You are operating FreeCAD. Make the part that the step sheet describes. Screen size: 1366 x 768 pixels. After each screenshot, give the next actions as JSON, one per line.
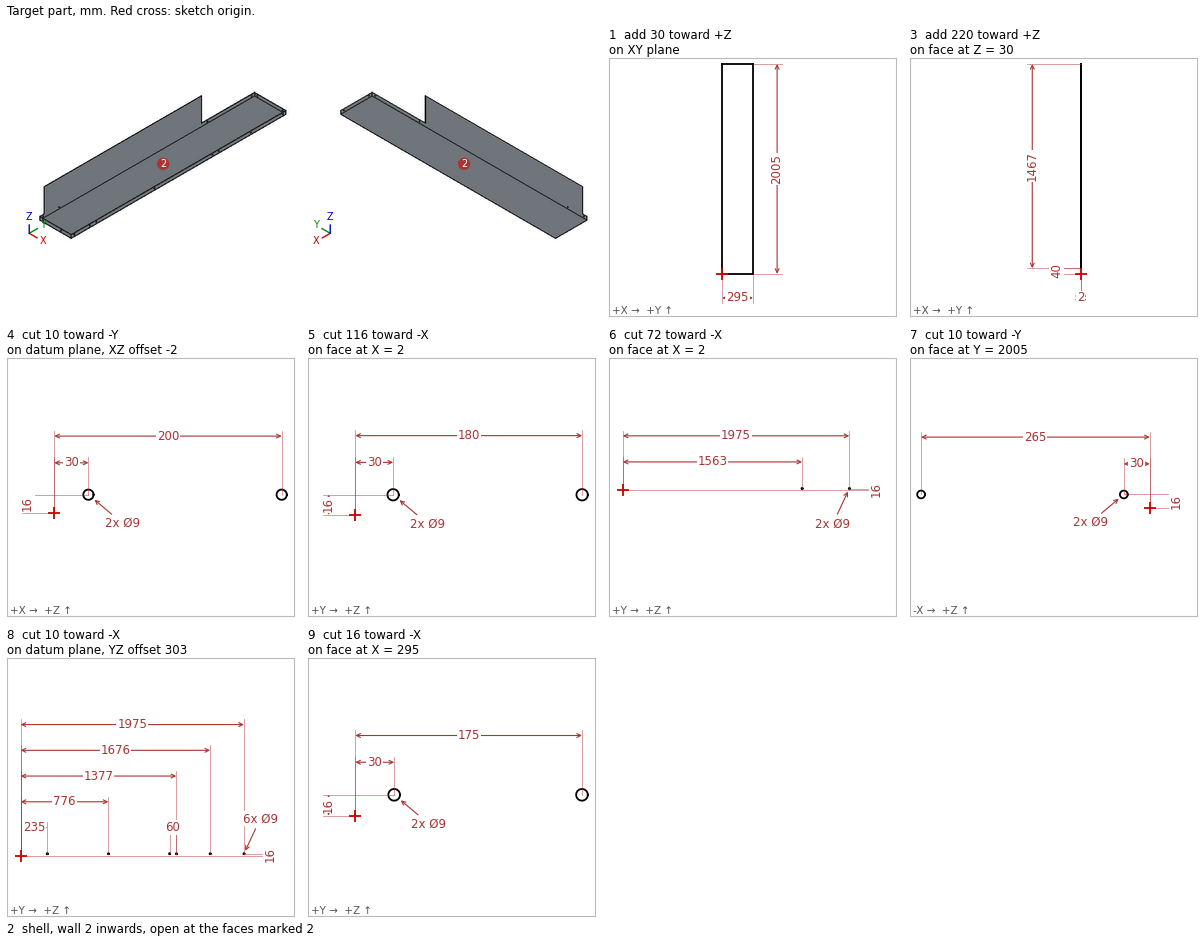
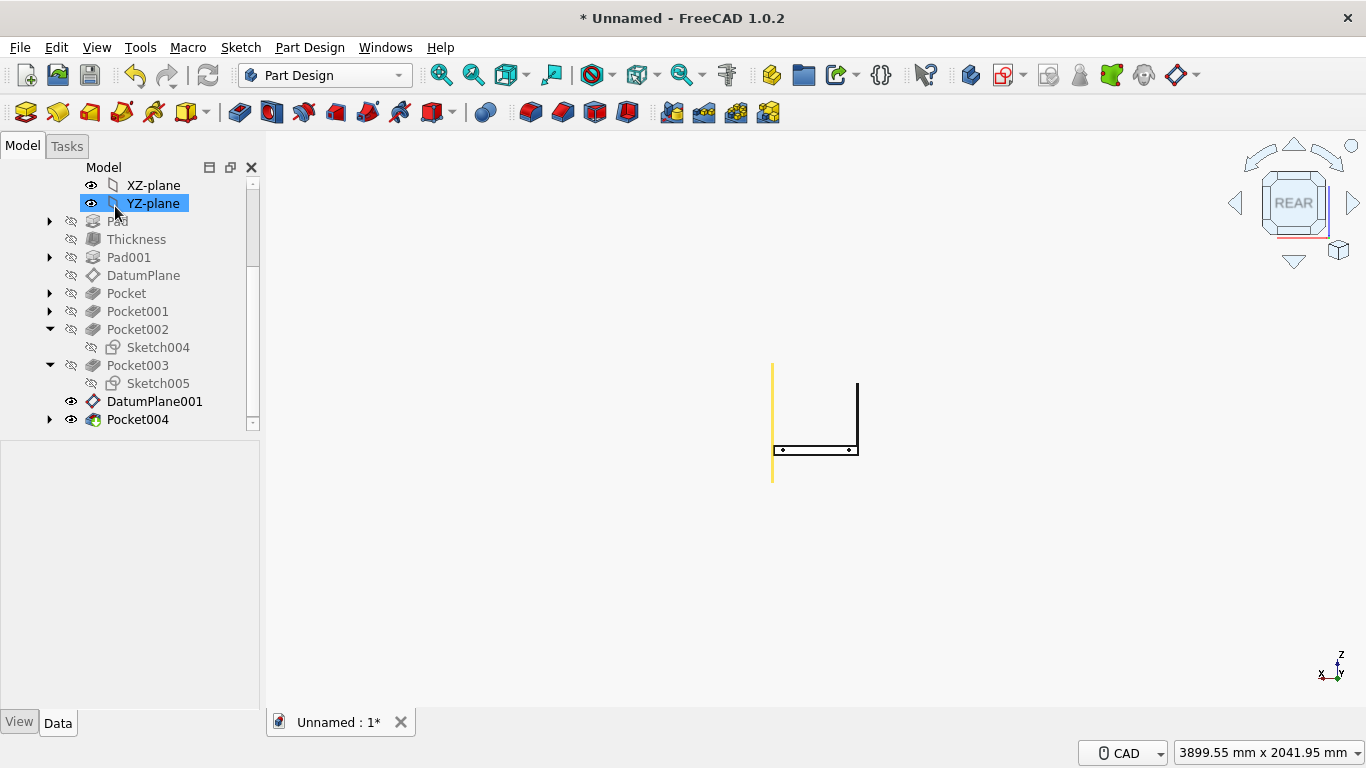
{"action": "left_click", "coordinate": [116, 401]}
{"action": "key", "text": "space"}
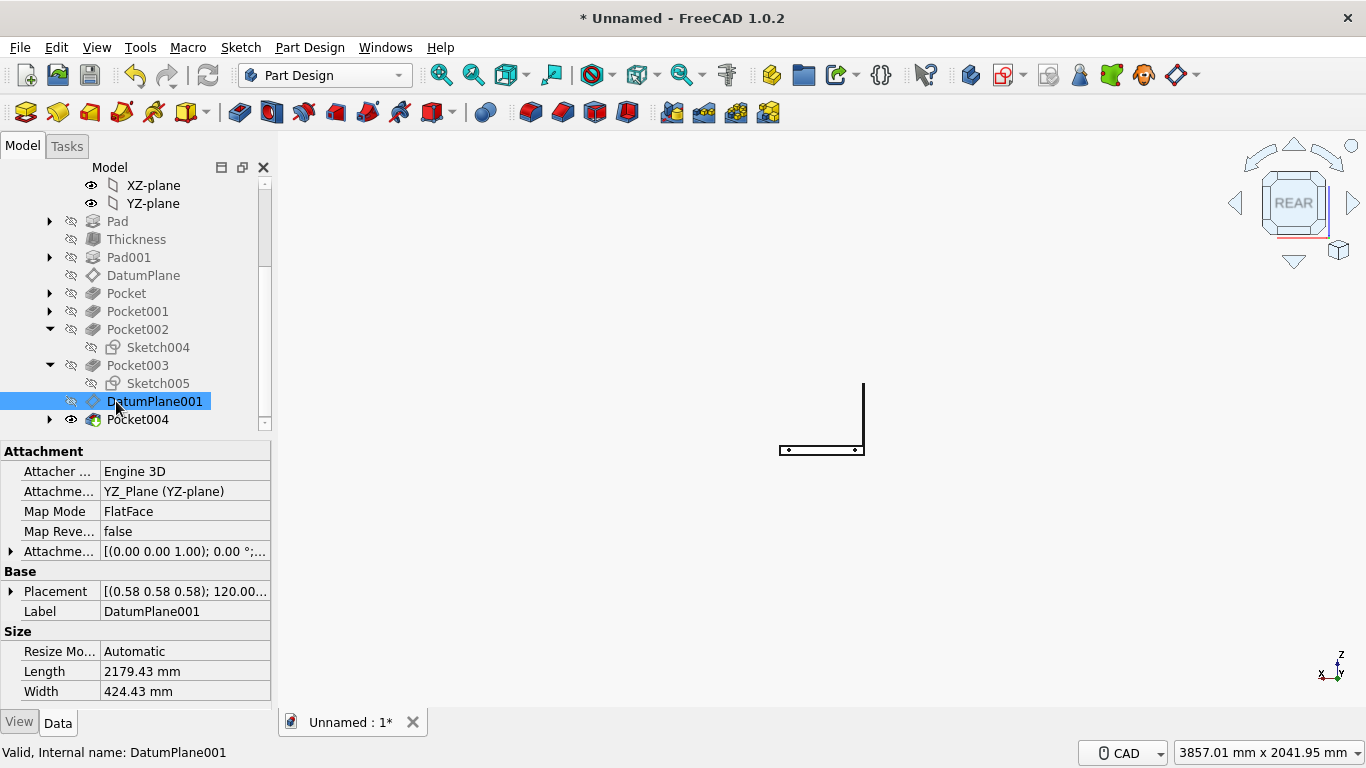
{"action": "key", "text": "v f"}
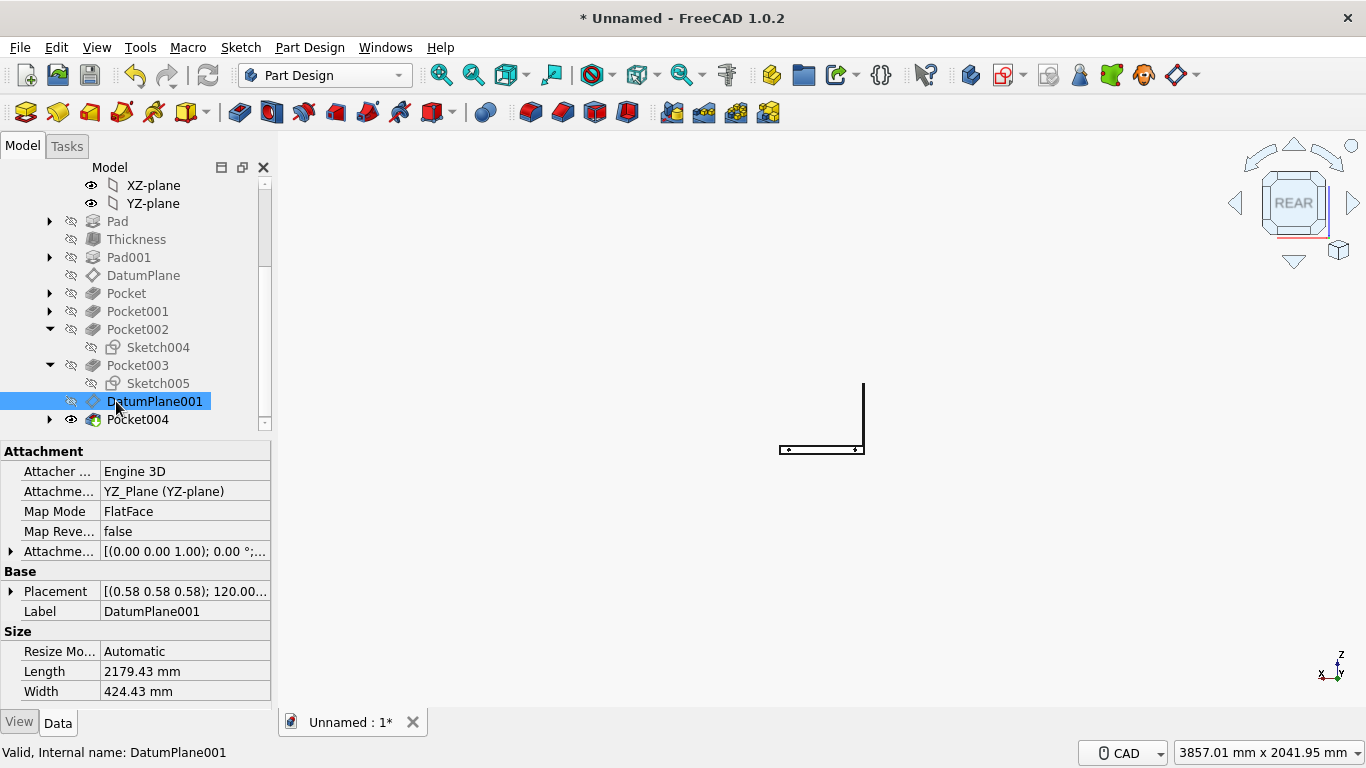
{"action": "key", "text": "0"}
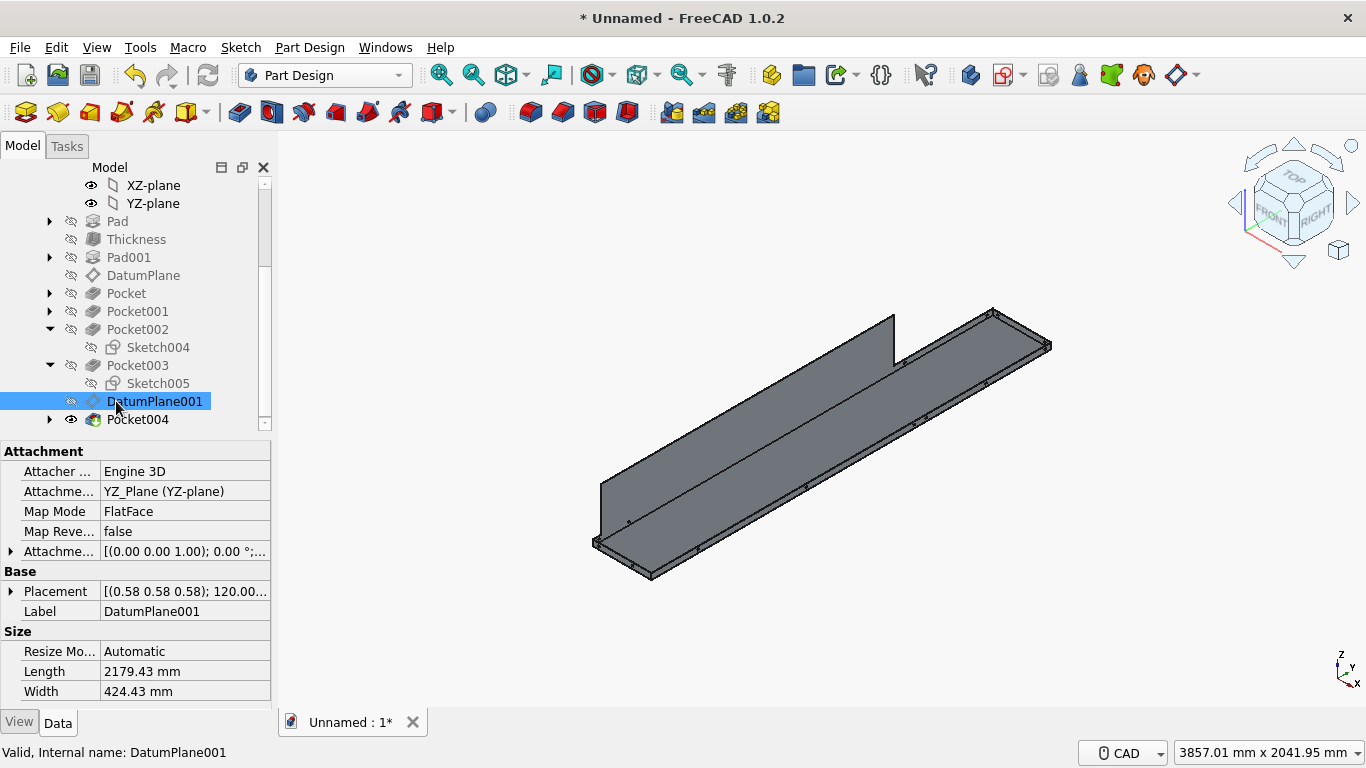
{"action": "scroll", "coordinate": [1023, 361], "scroll_direction": "up", "scroll_amount": 6}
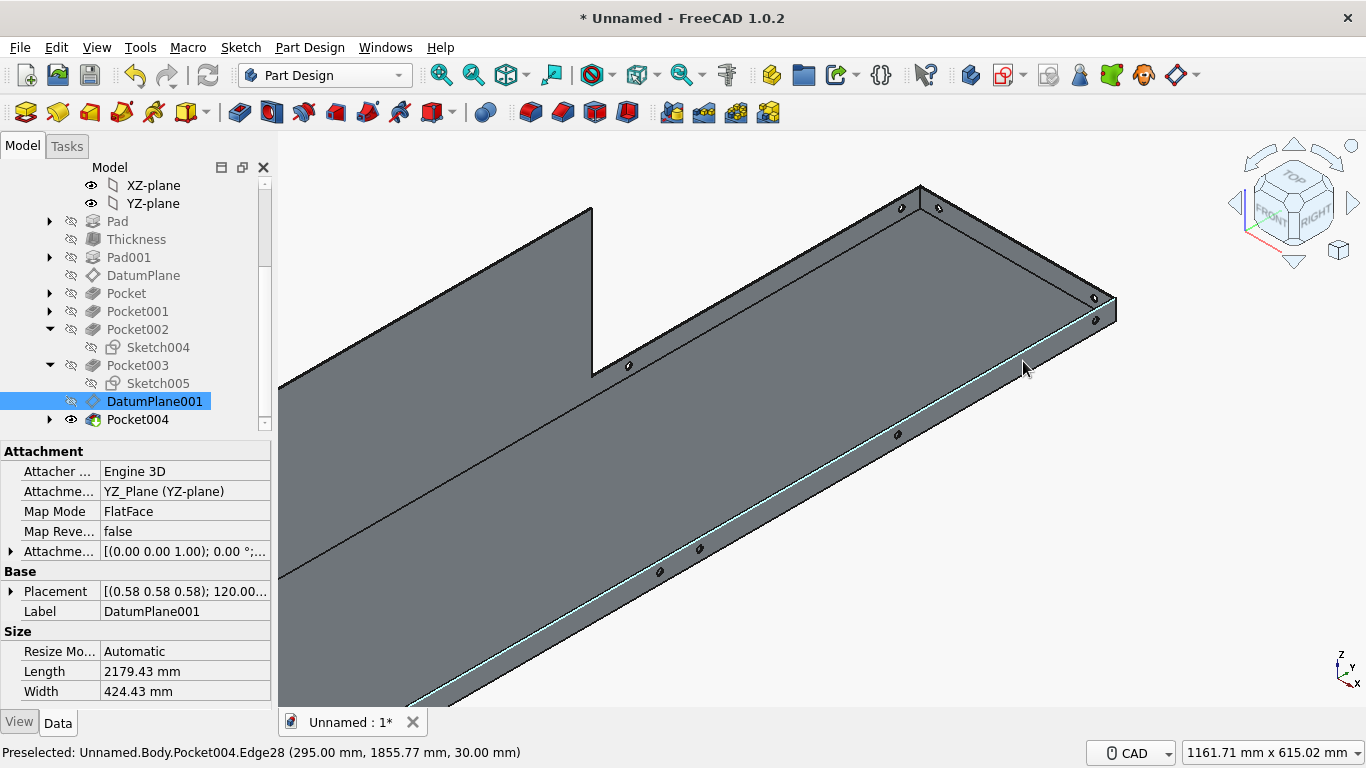
{"action": "left_click", "coordinate": [1021, 364]}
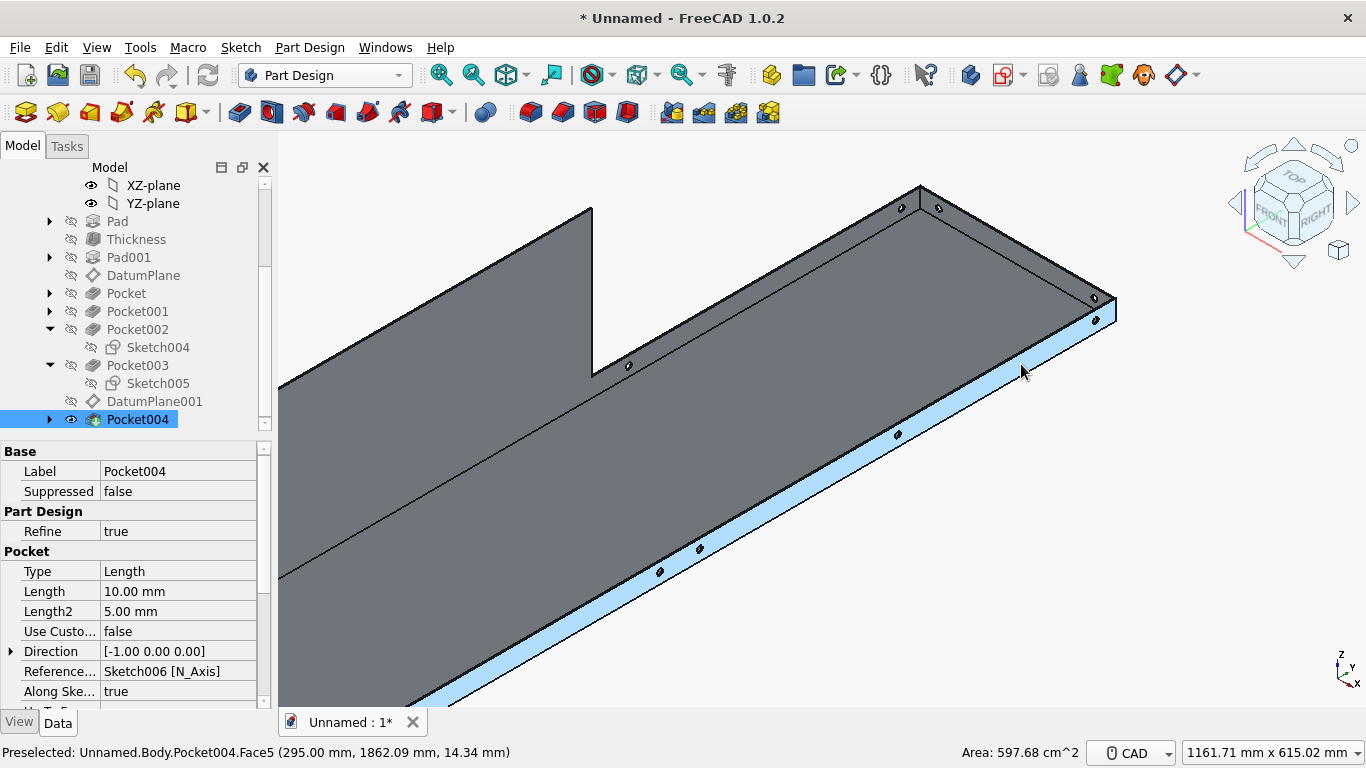
{"action": "left_click", "coordinate": [1004, 76]}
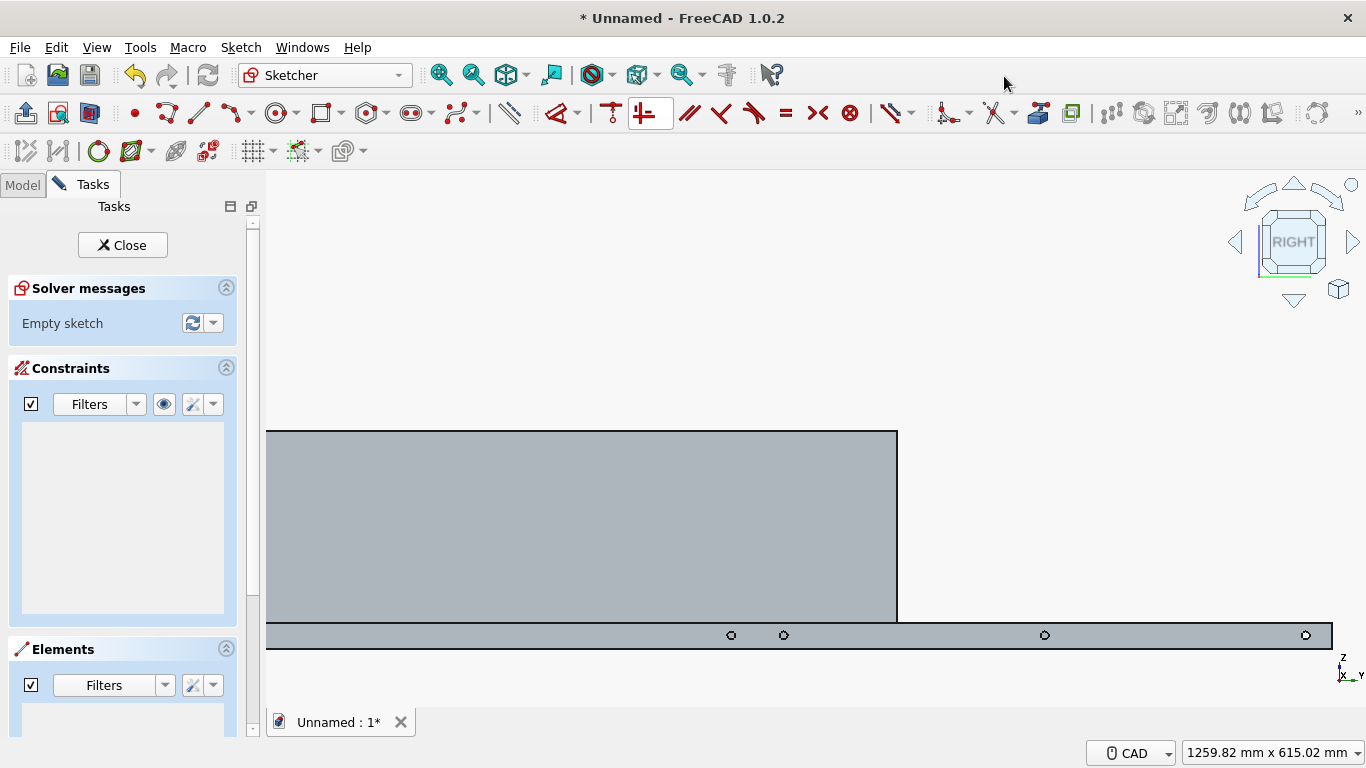
{"action": "scroll", "coordinate": [748, 438], "scroll_direction": "down", "scroll_amount": 5}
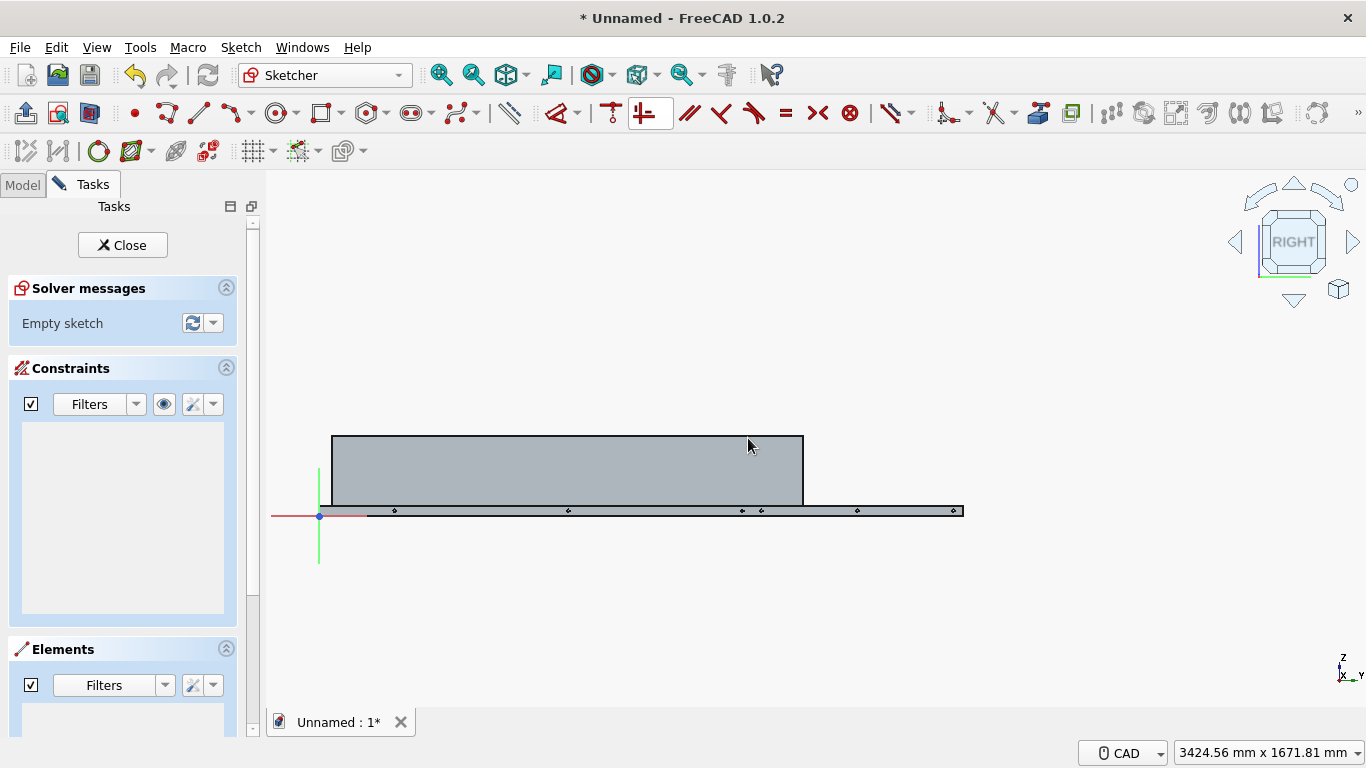
{"action": "scroll", "coordinate": [308, 520], "scroll_direction": "up", "scroll_amount": 12}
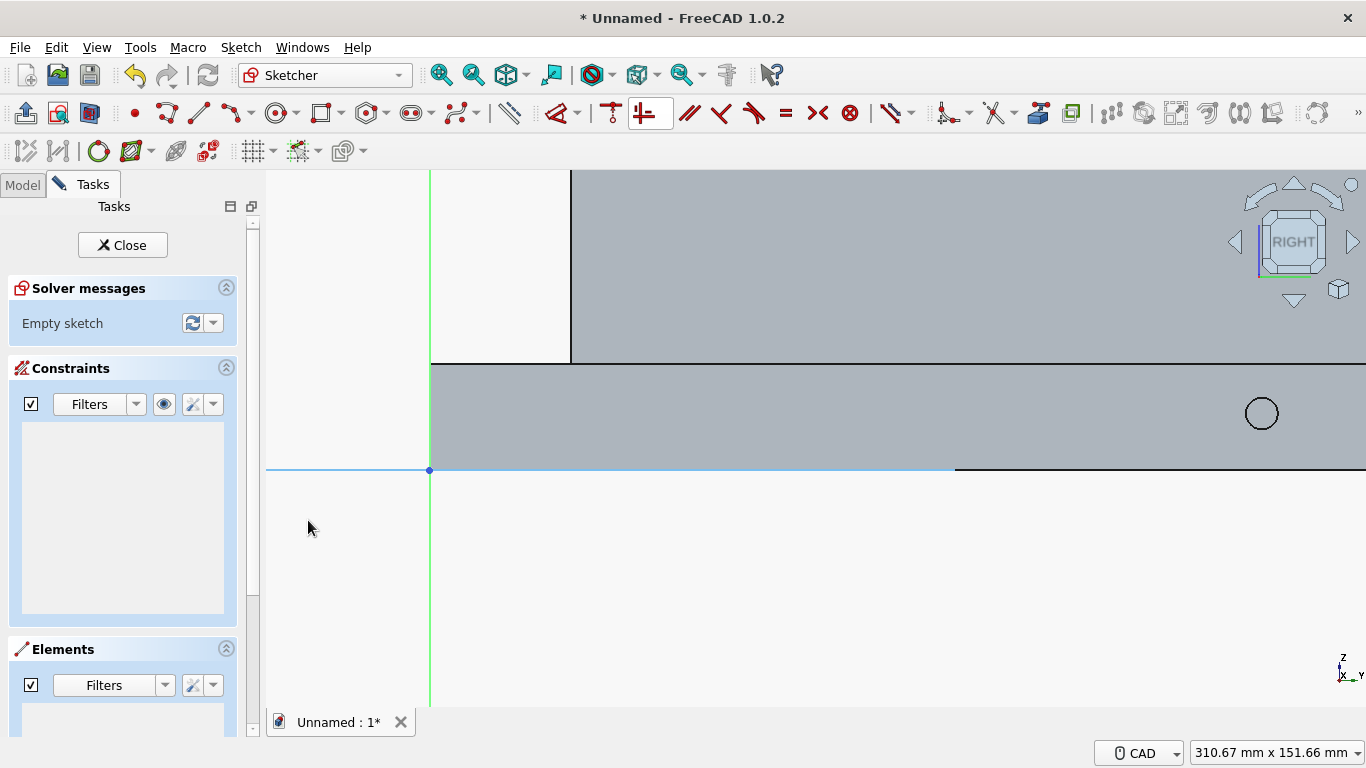
{"action": "left_click", "coordinate": [276, 114]}